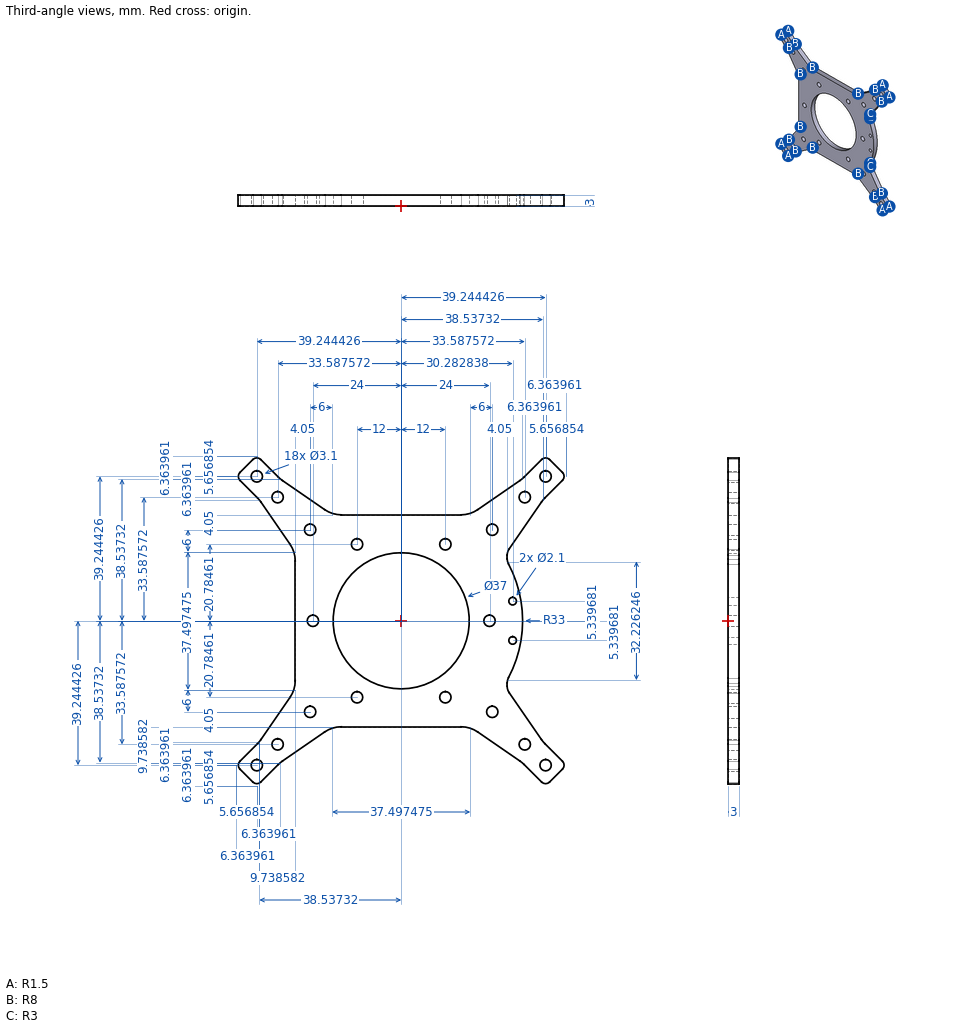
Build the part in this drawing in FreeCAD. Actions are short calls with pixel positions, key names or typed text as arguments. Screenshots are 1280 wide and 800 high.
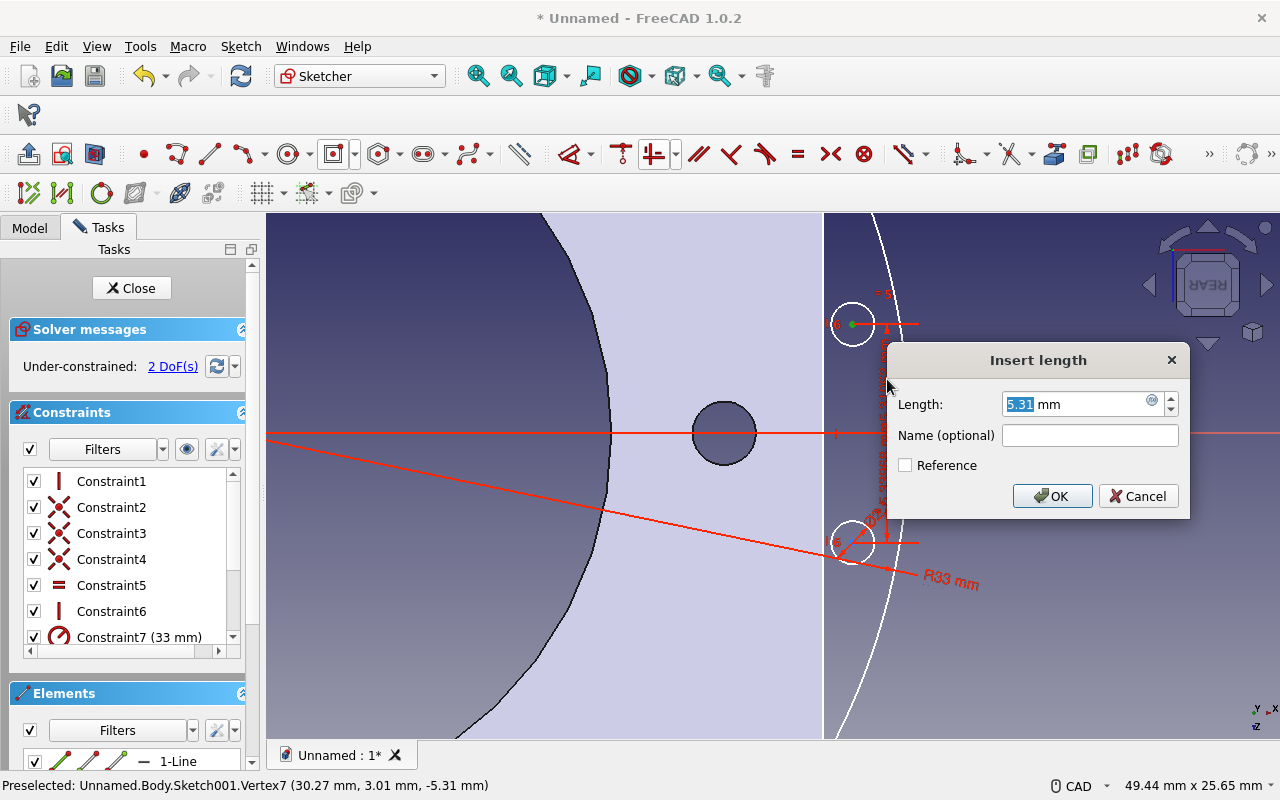
text(5.339681)
key(Return)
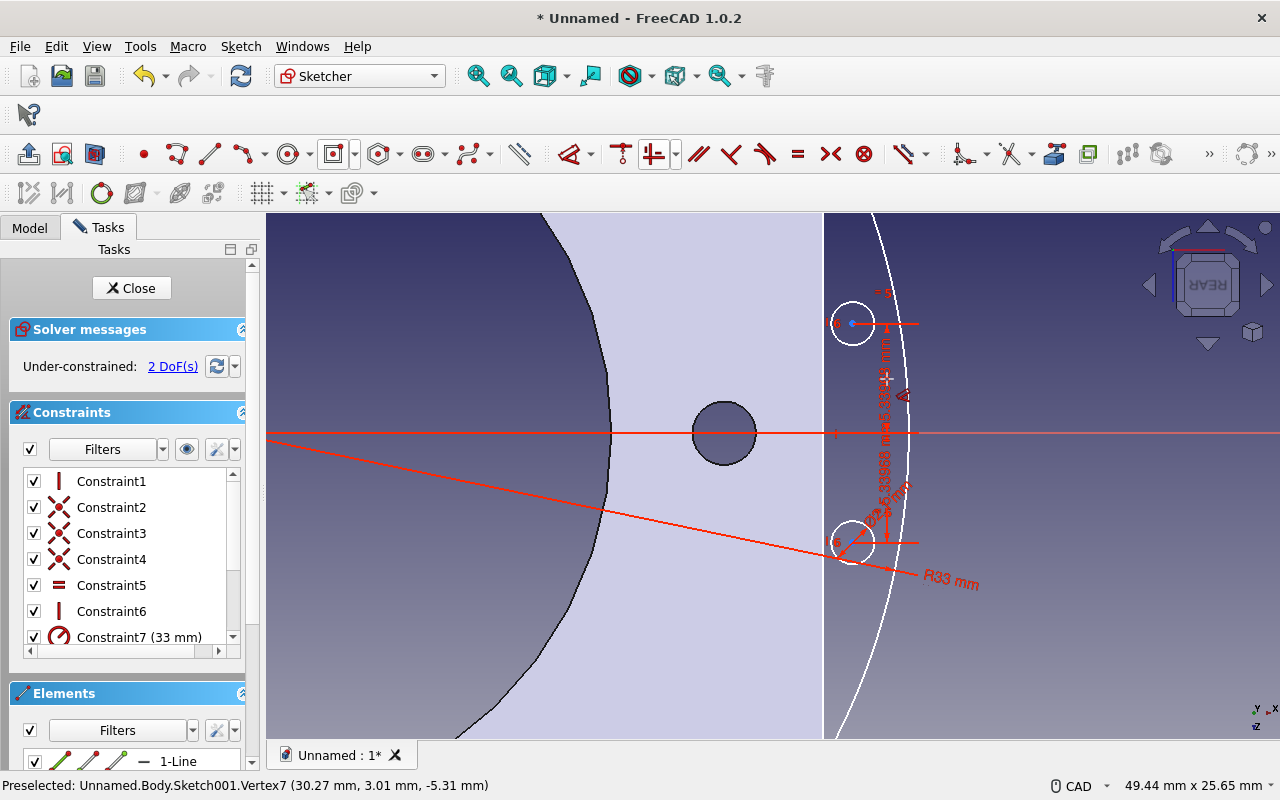
click(823, 301)
click(857, 584)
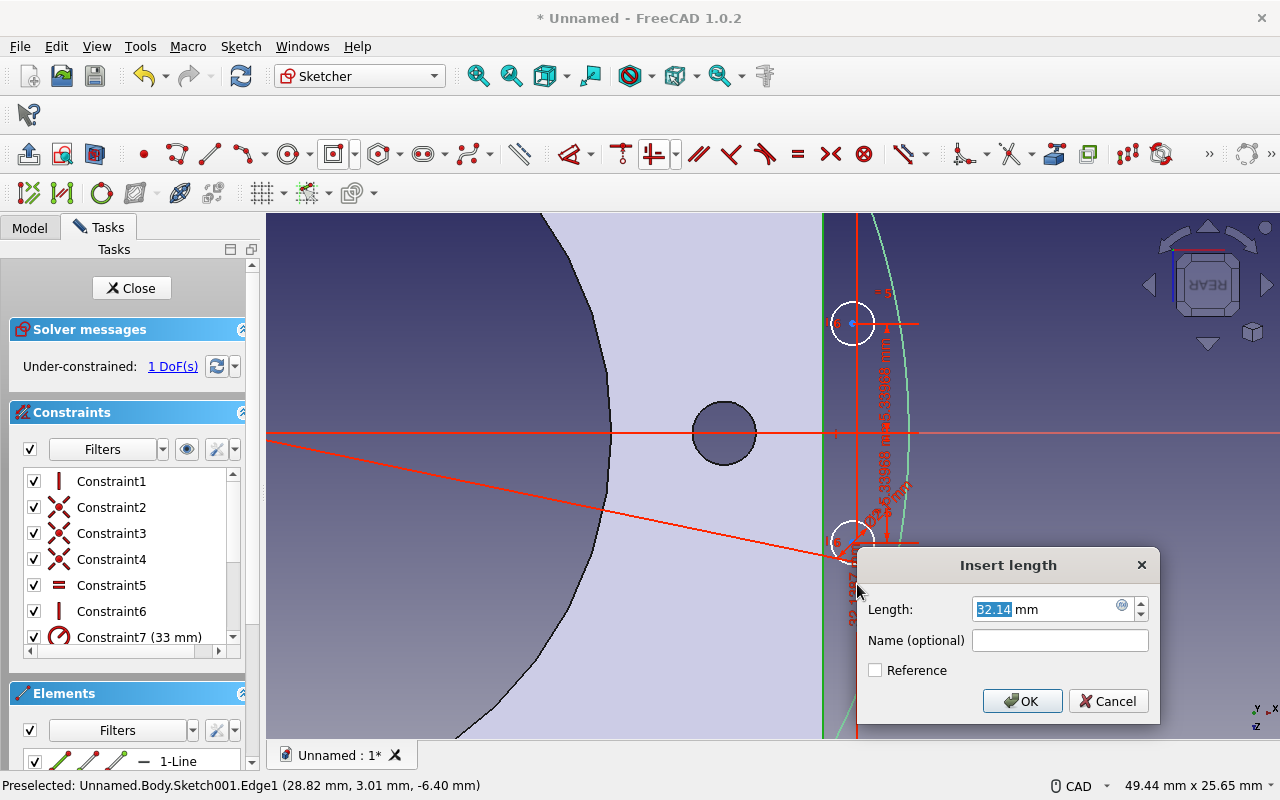
text(32.226246)
key(Return)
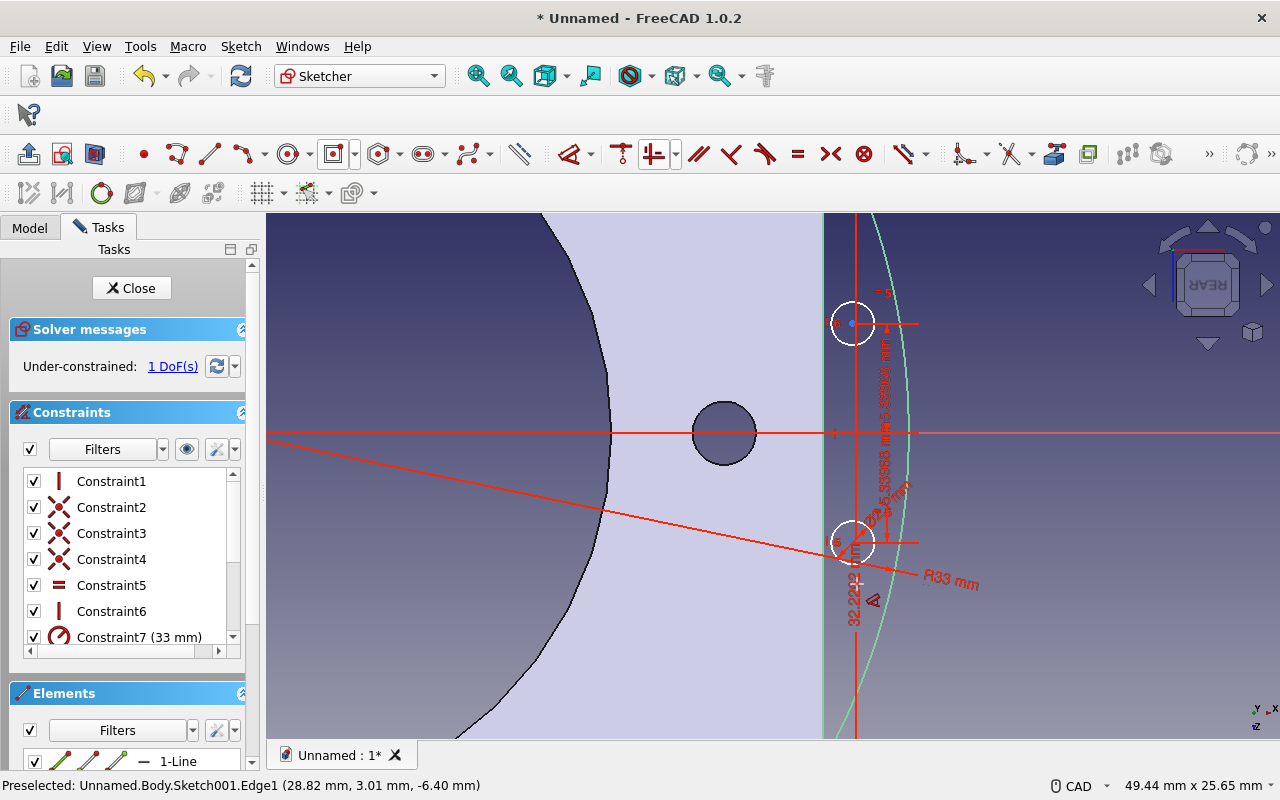
click(853, 543)
click(573, 577)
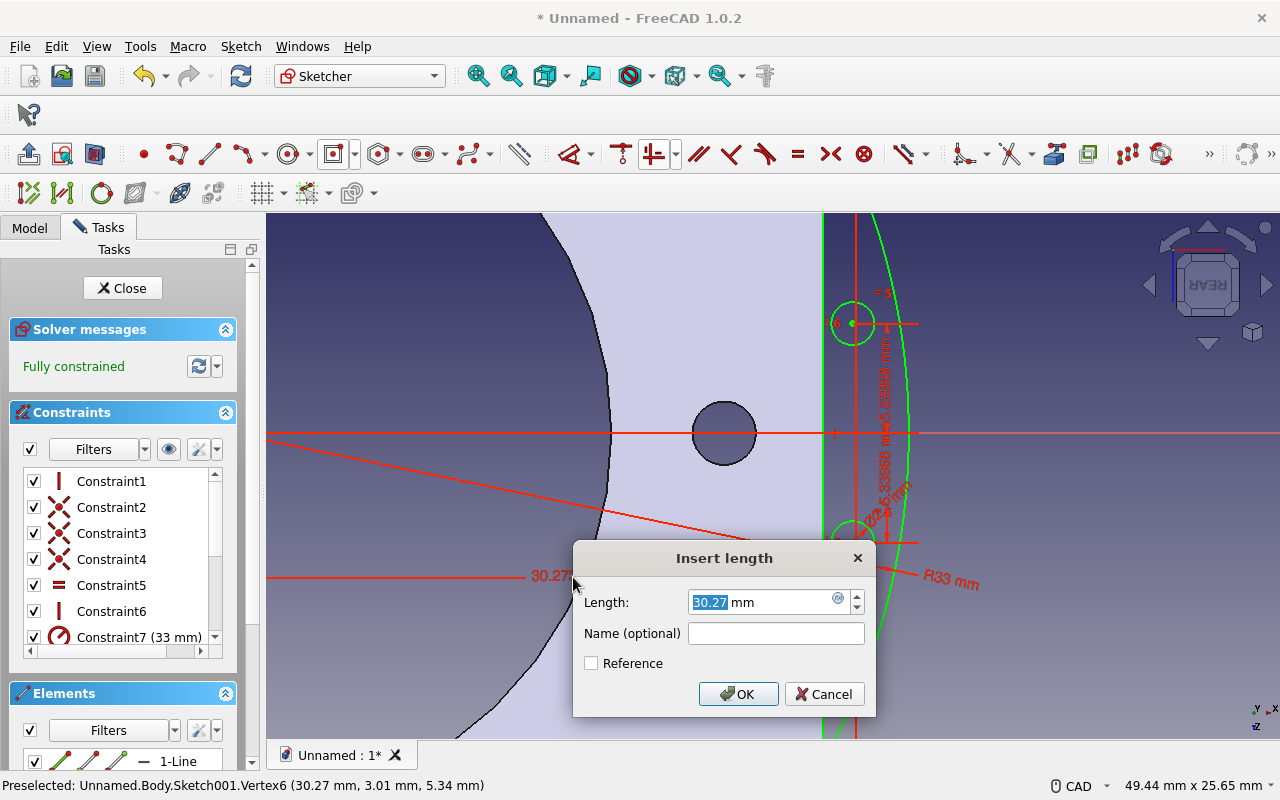
text(30.282838)
key(Return)
key(Escape)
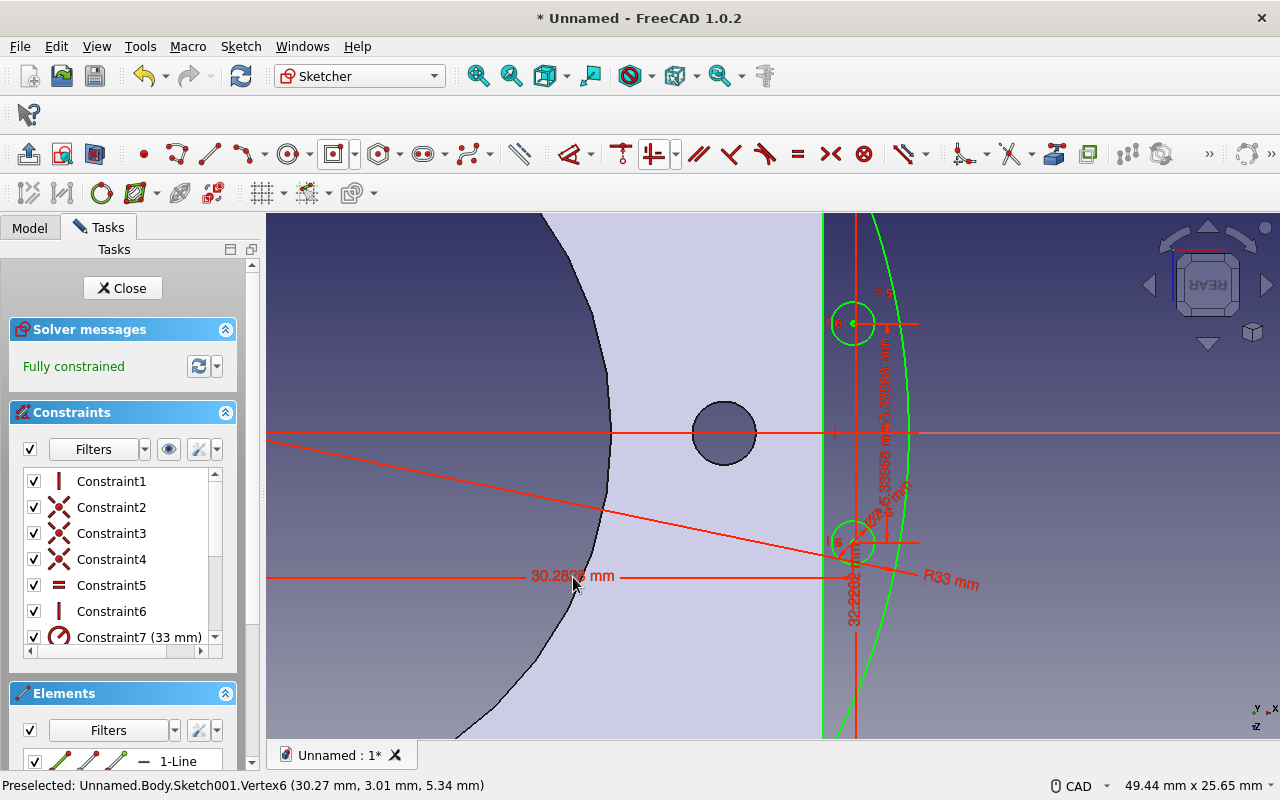
click(123, 288)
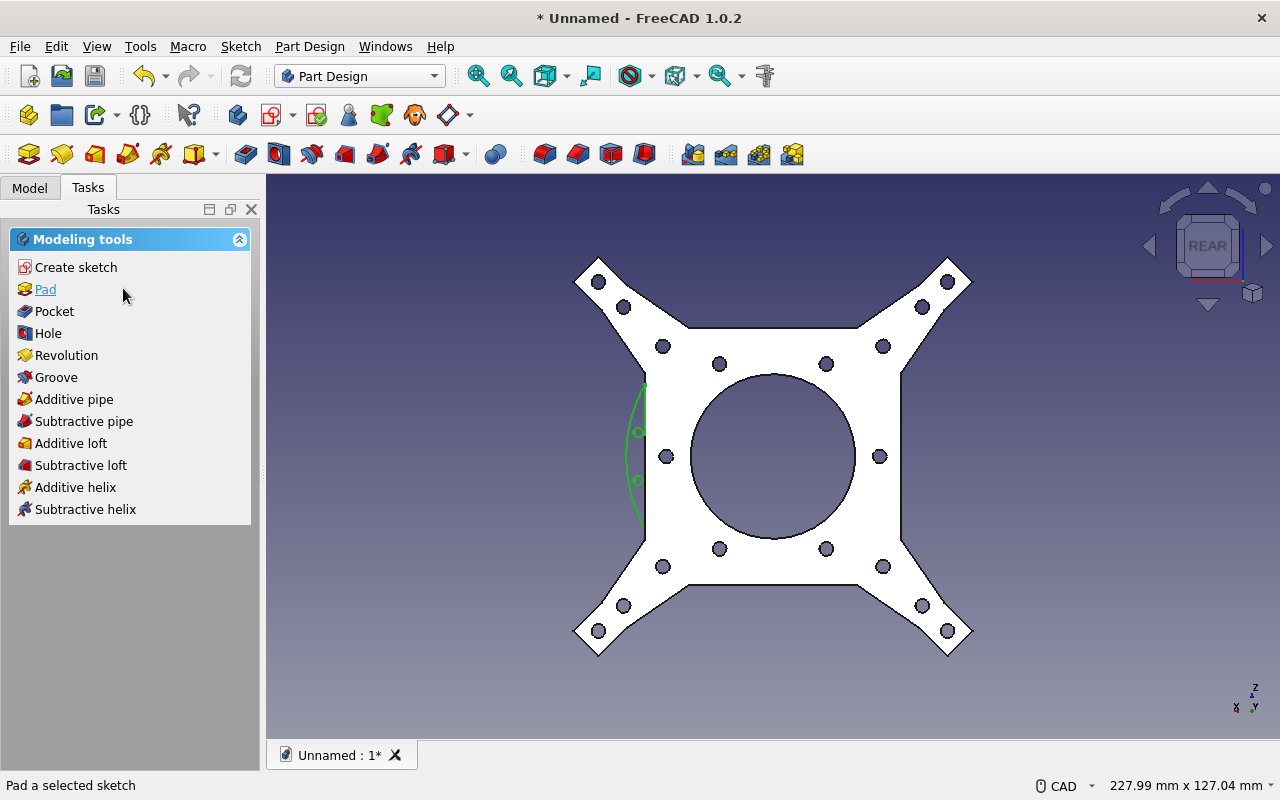
click(29, 154)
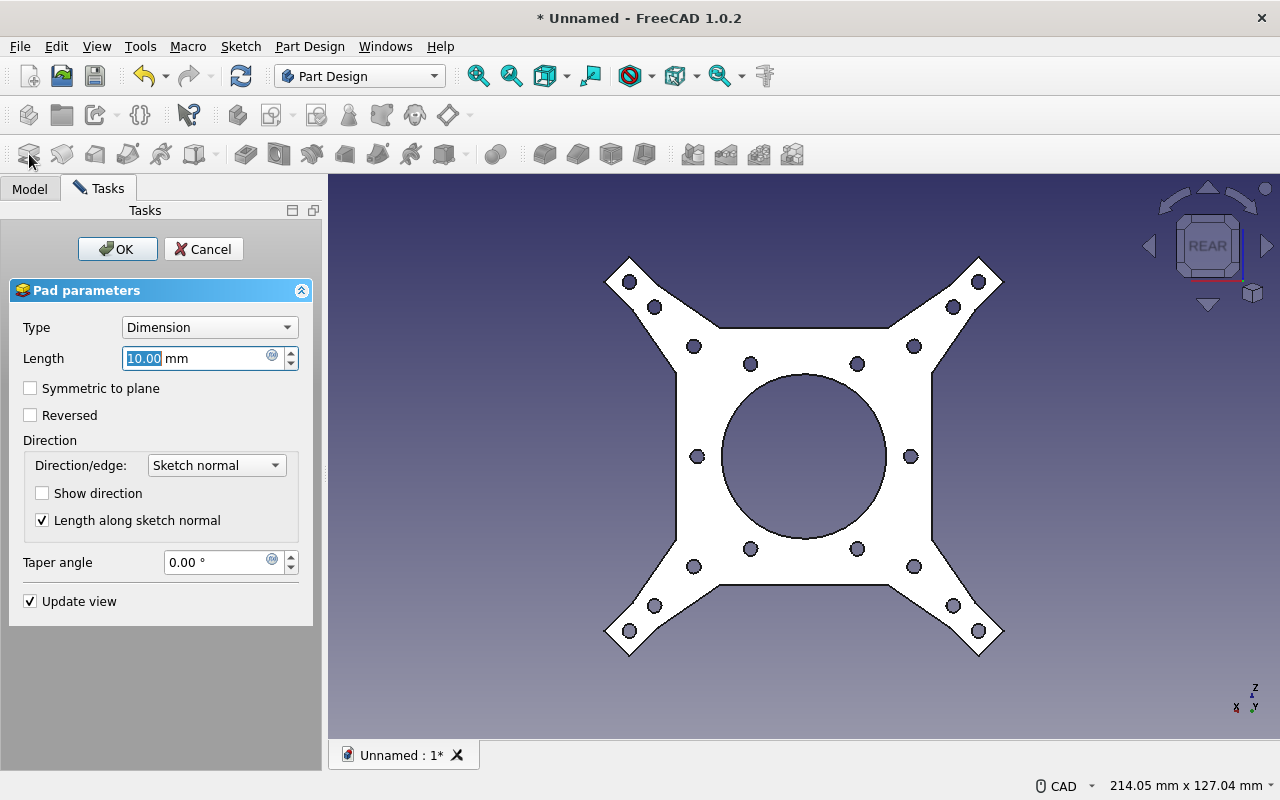
text(3)
key(Tab)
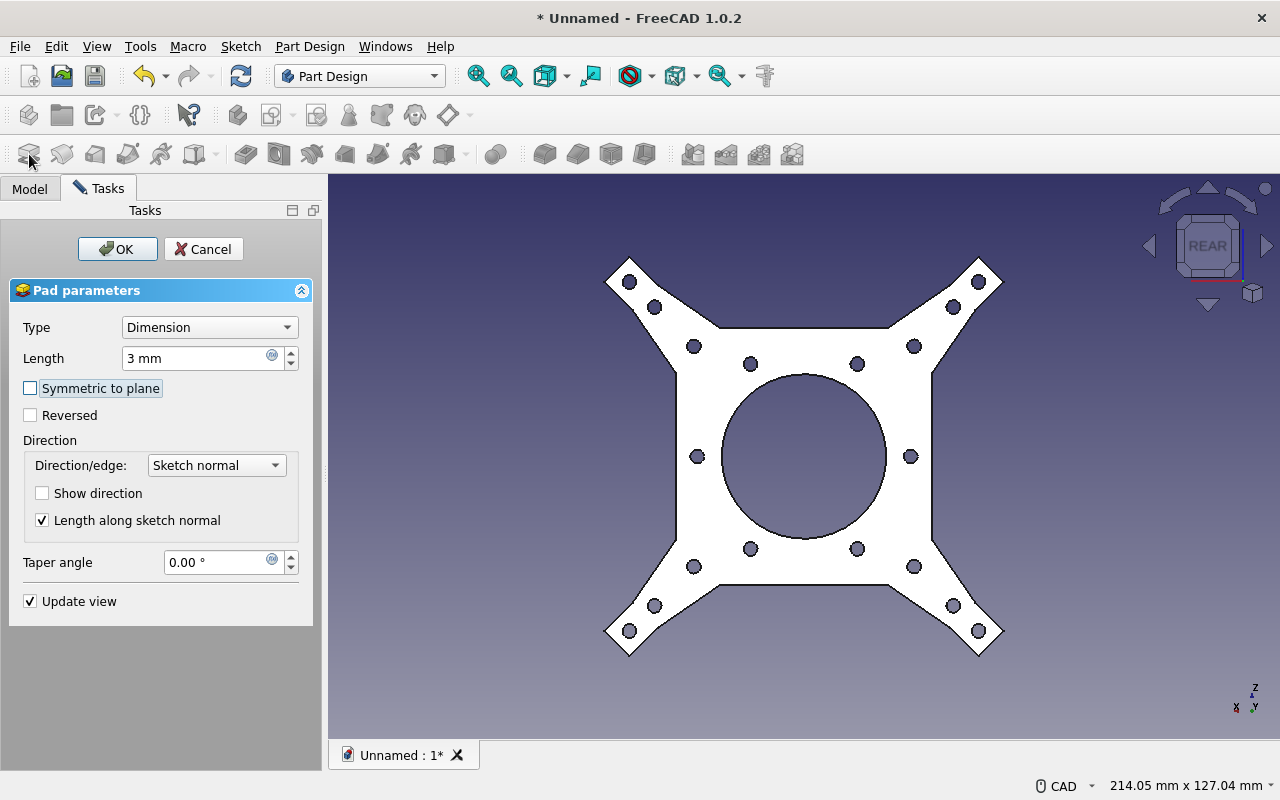
click(31, 415)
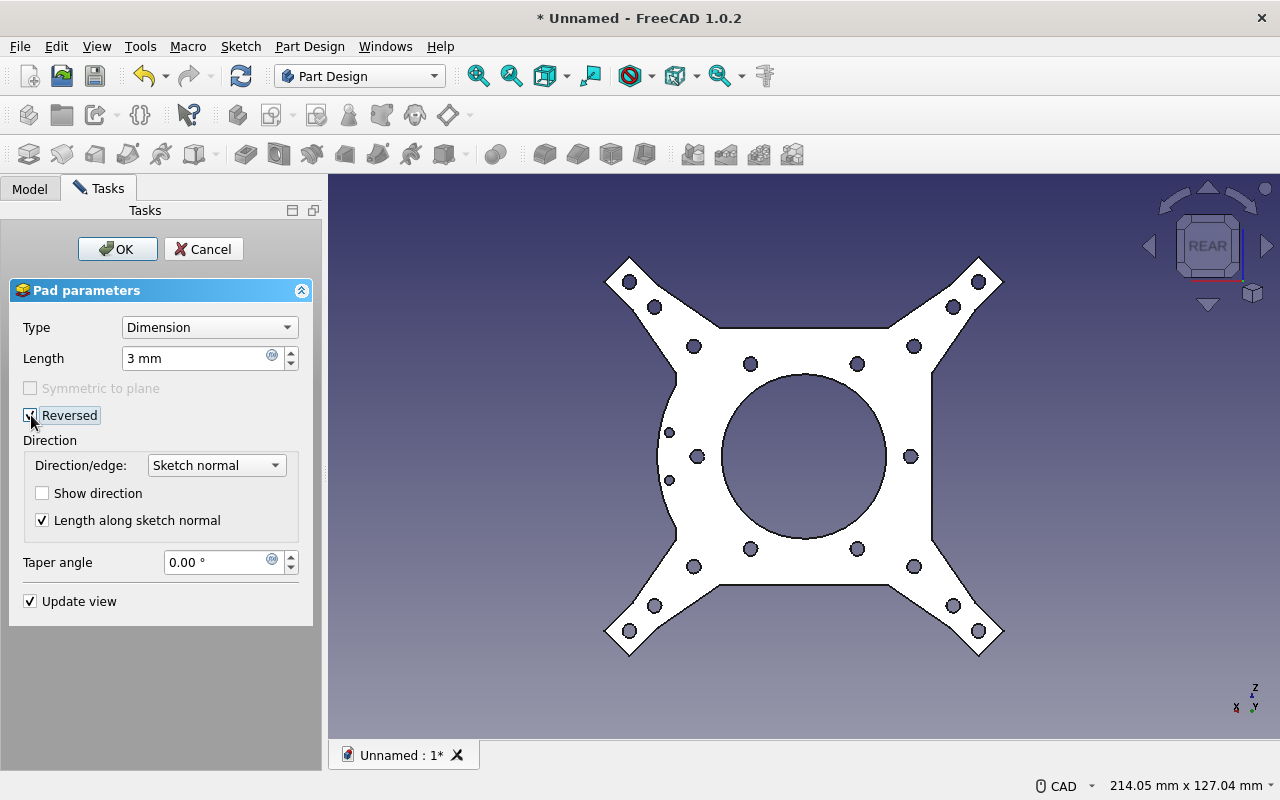
click(118, 249)